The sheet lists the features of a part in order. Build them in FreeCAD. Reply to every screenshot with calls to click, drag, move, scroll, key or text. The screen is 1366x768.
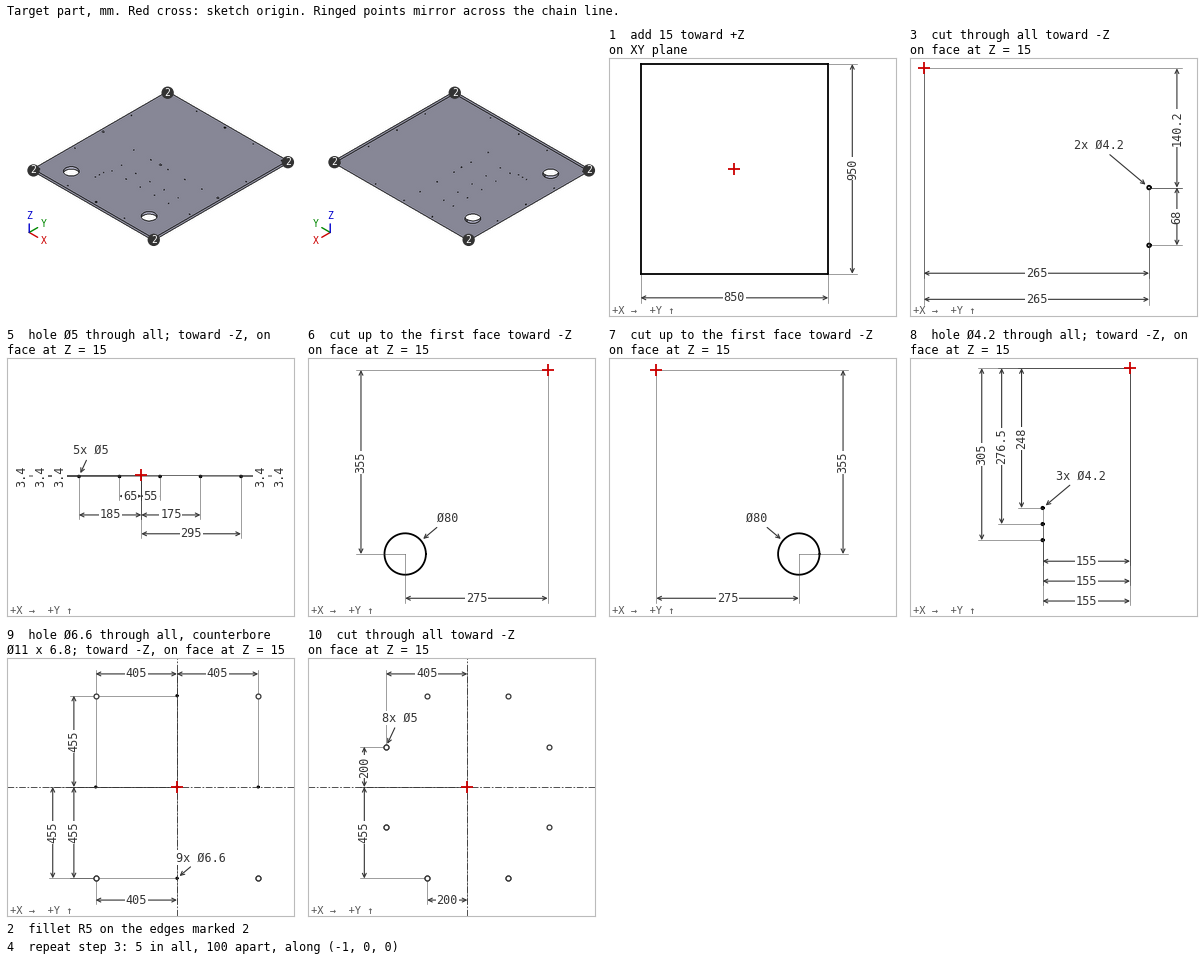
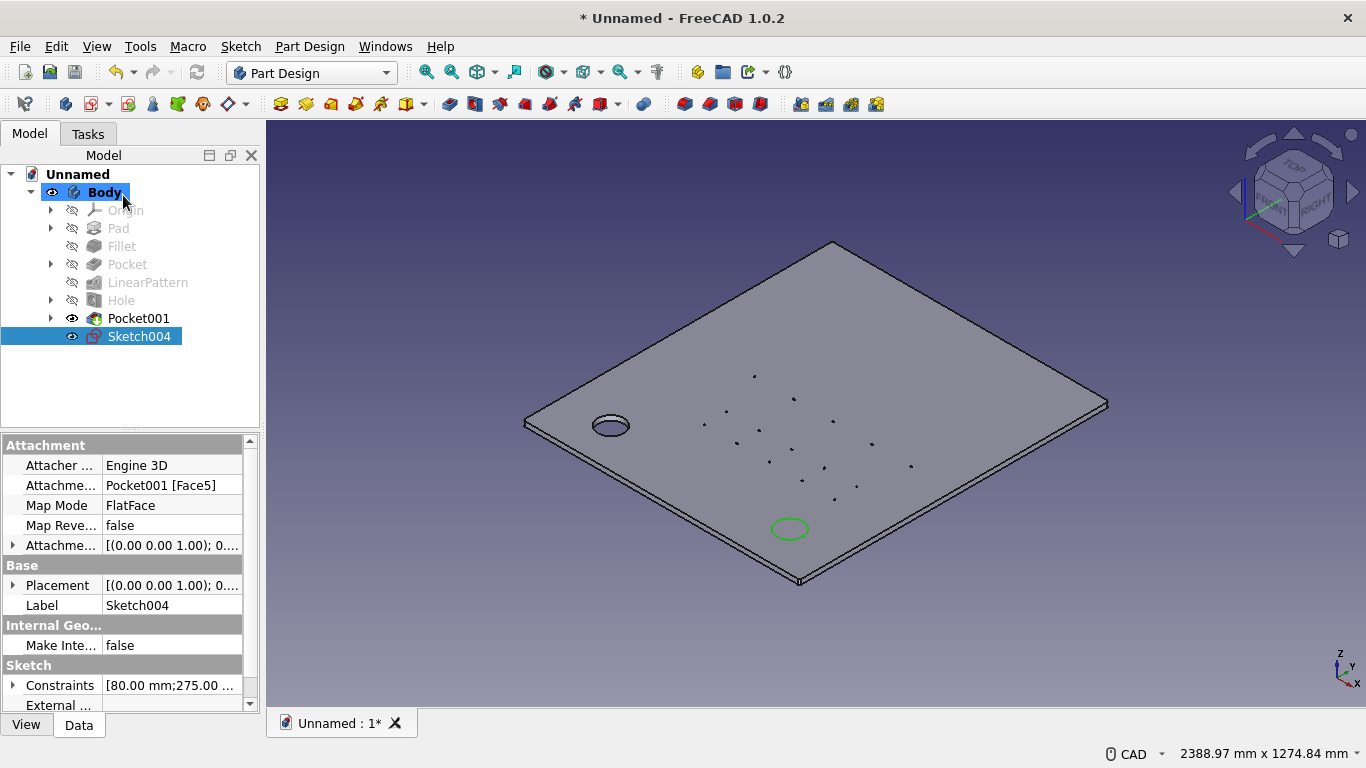
click(450, 104)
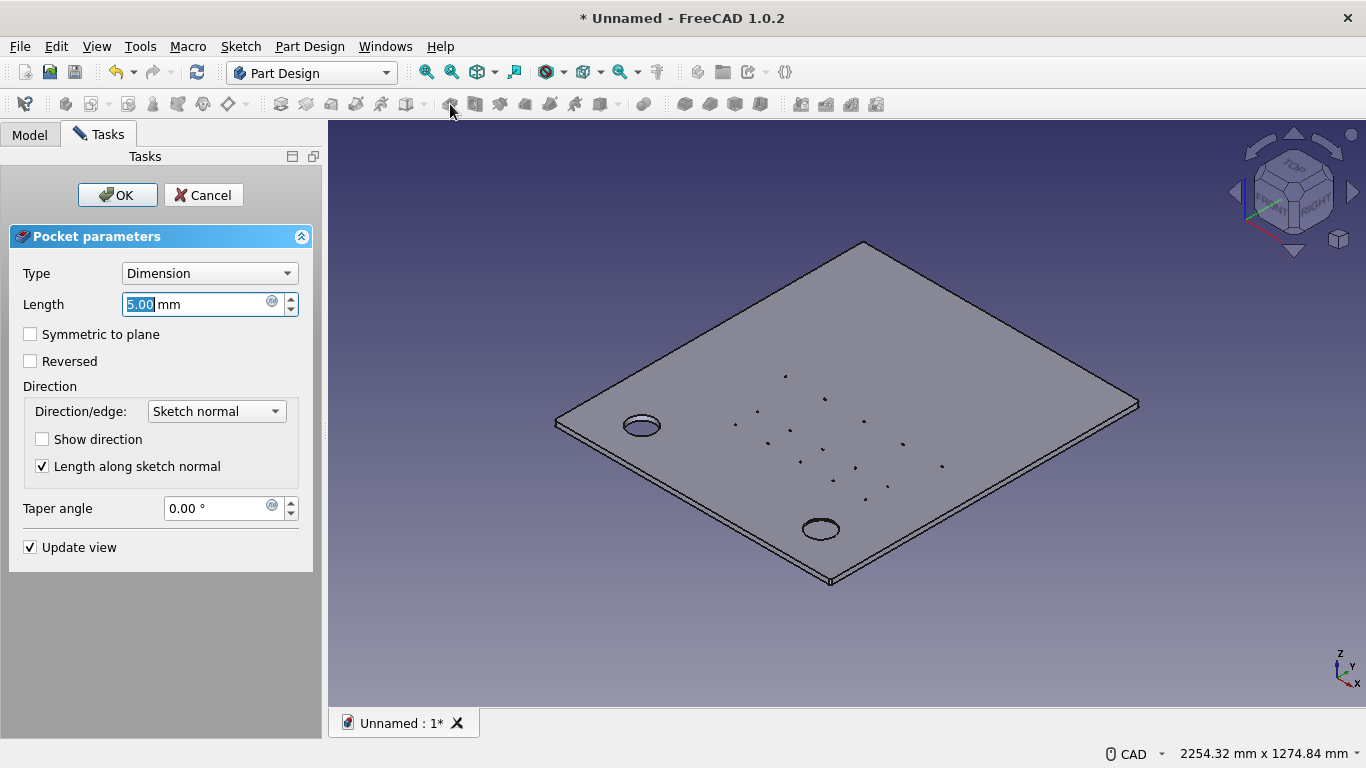
click(210, 274)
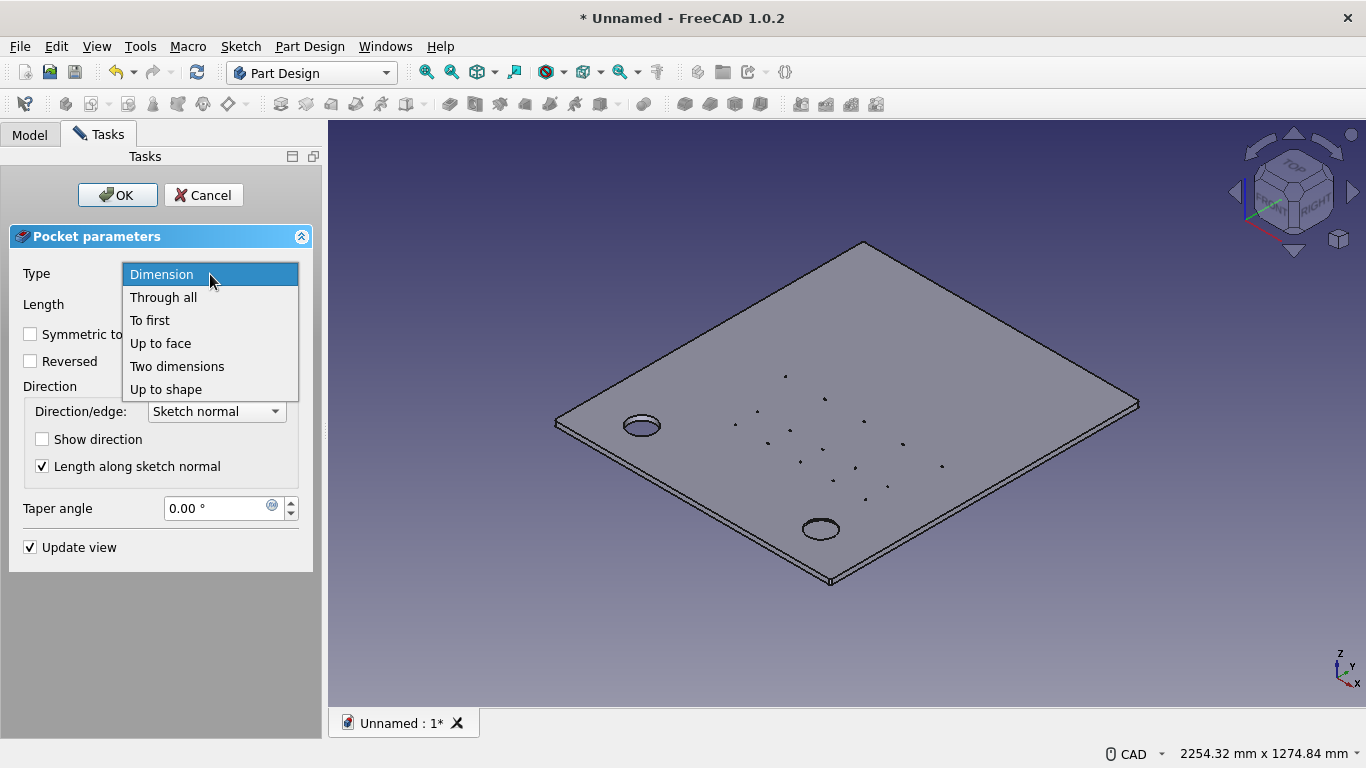
click(208, 320)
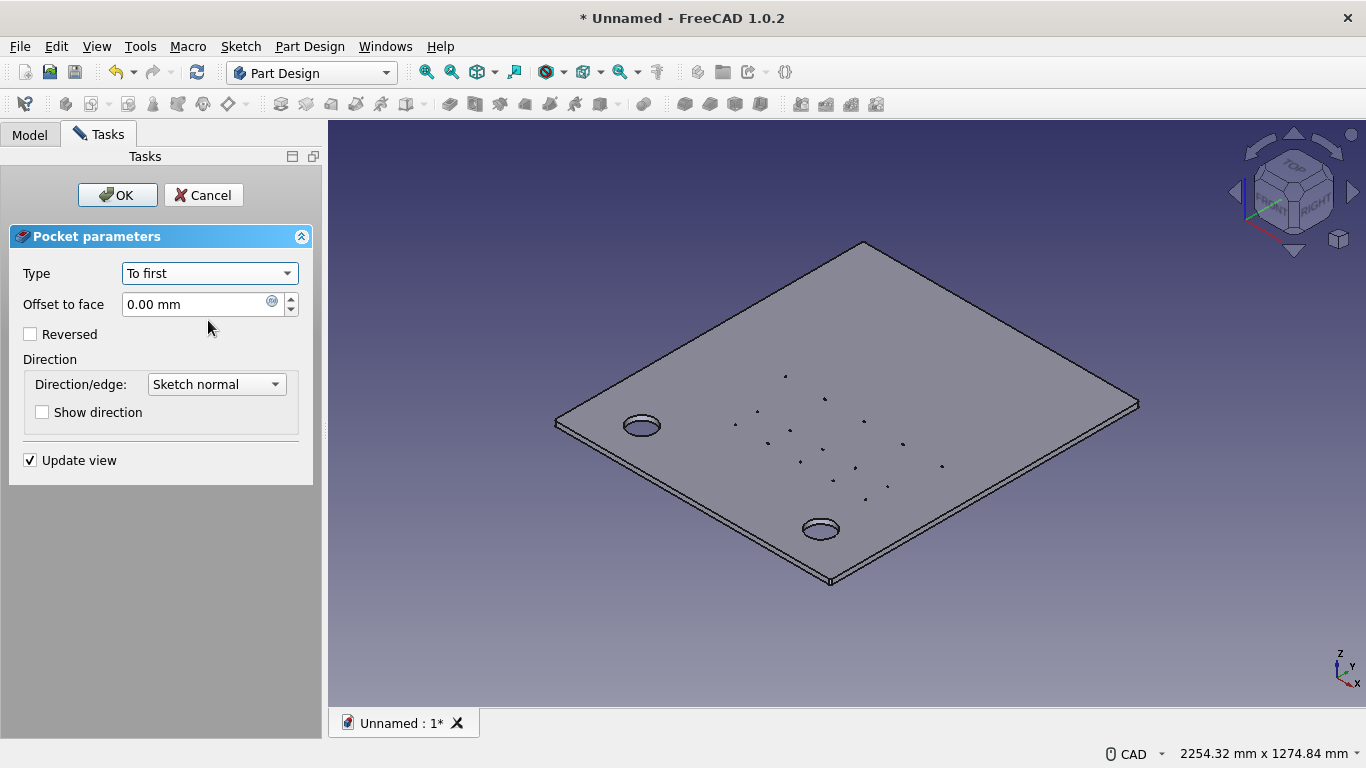
click(118, 195)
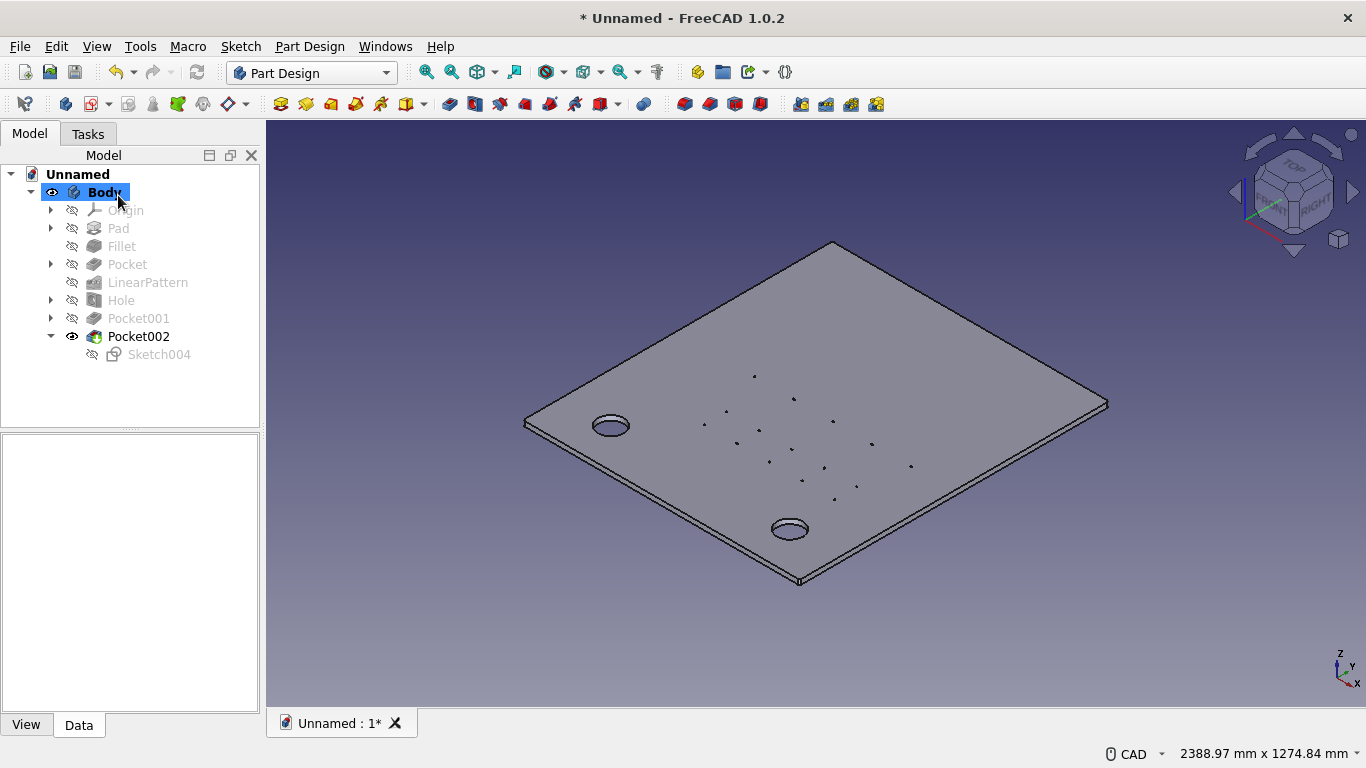
click(944, 381)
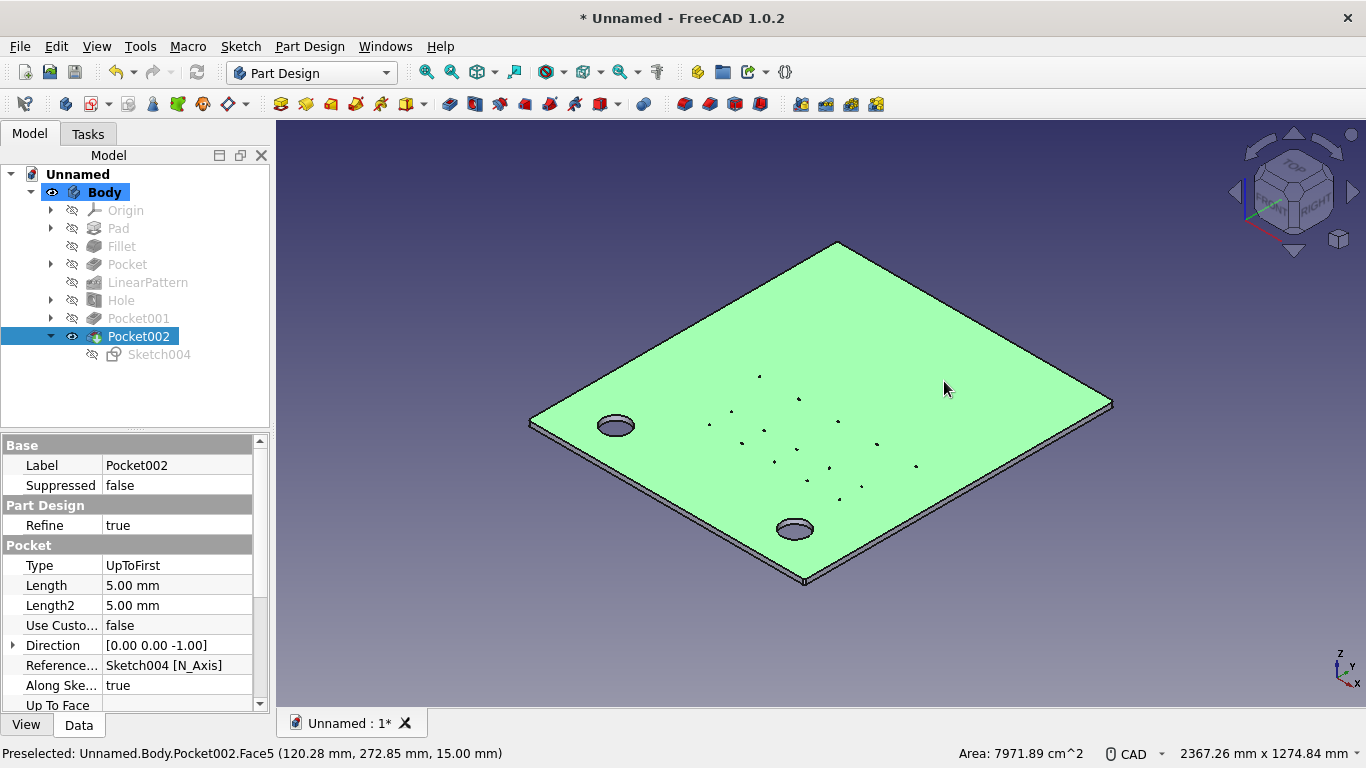
click(90, 104)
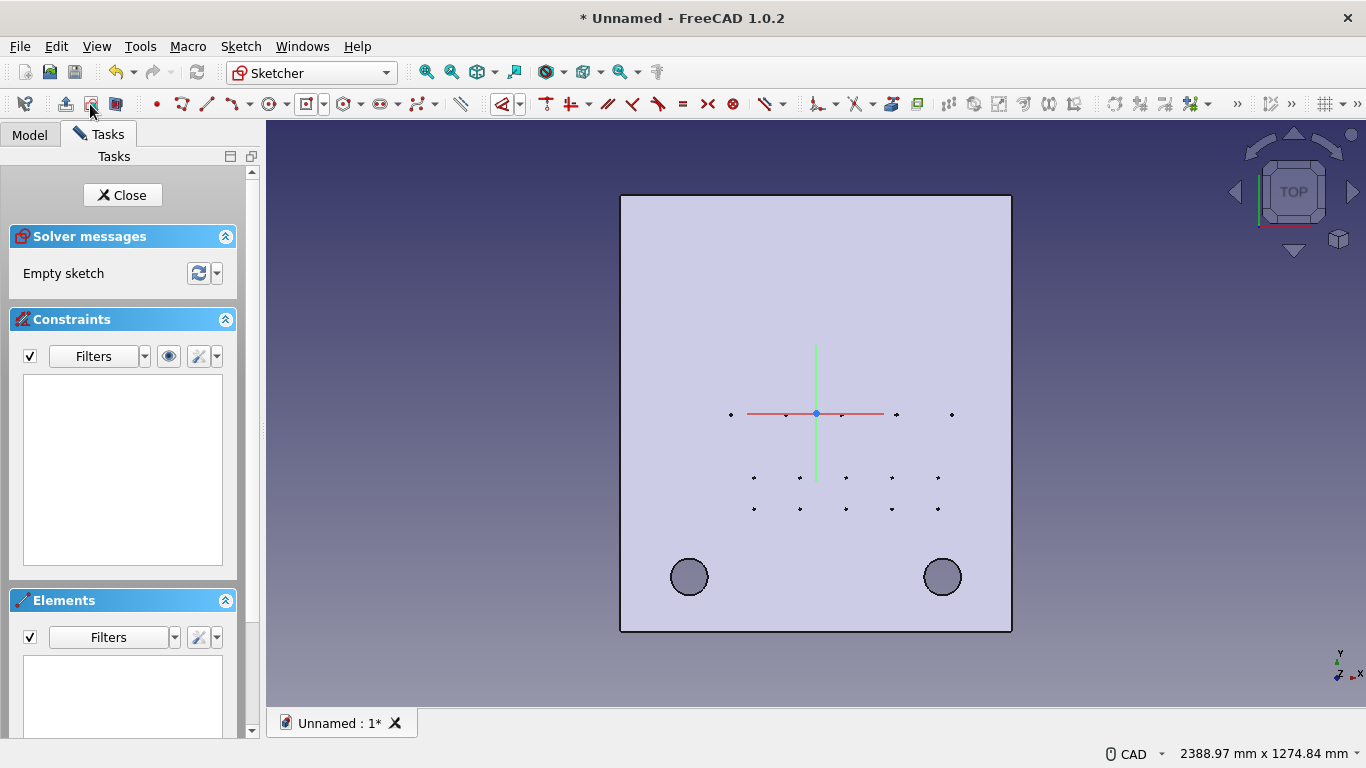
scroll(744, 551, up, 13)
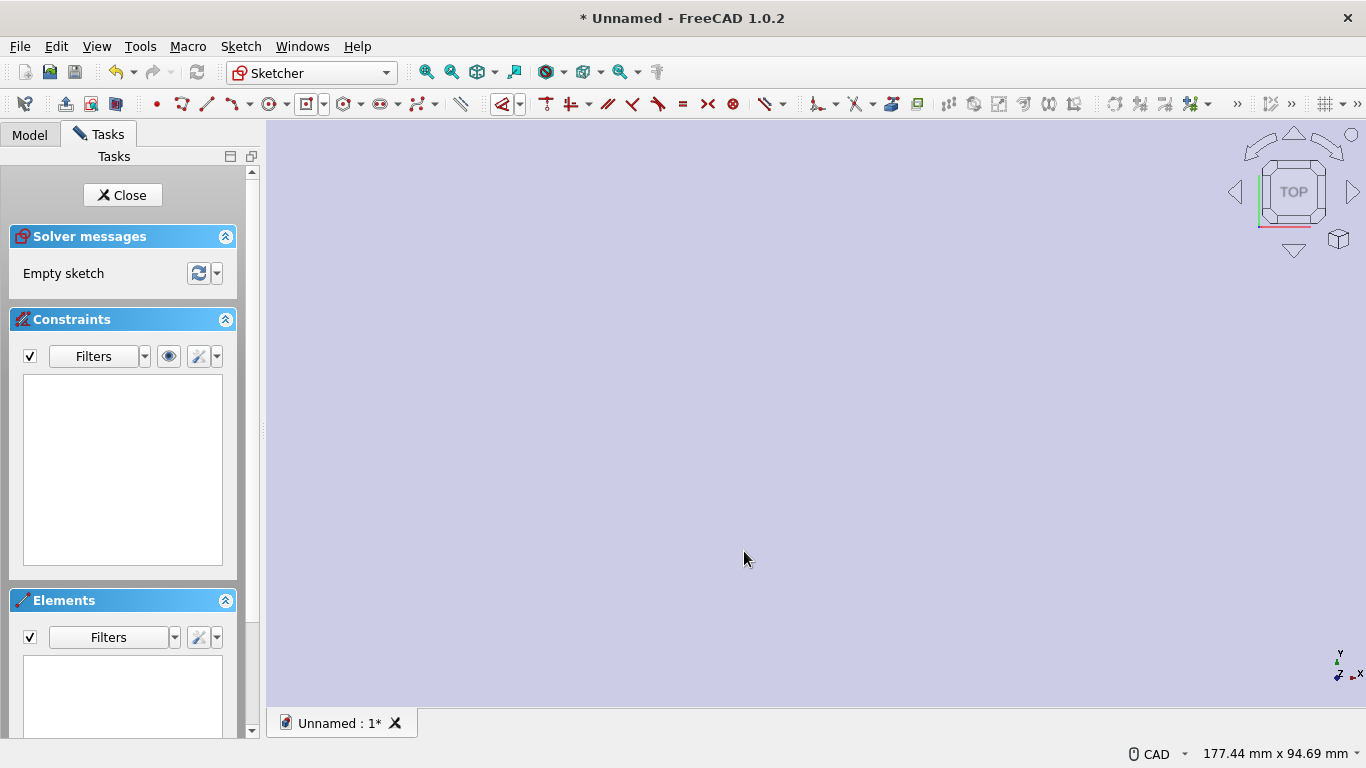
click(268, 104)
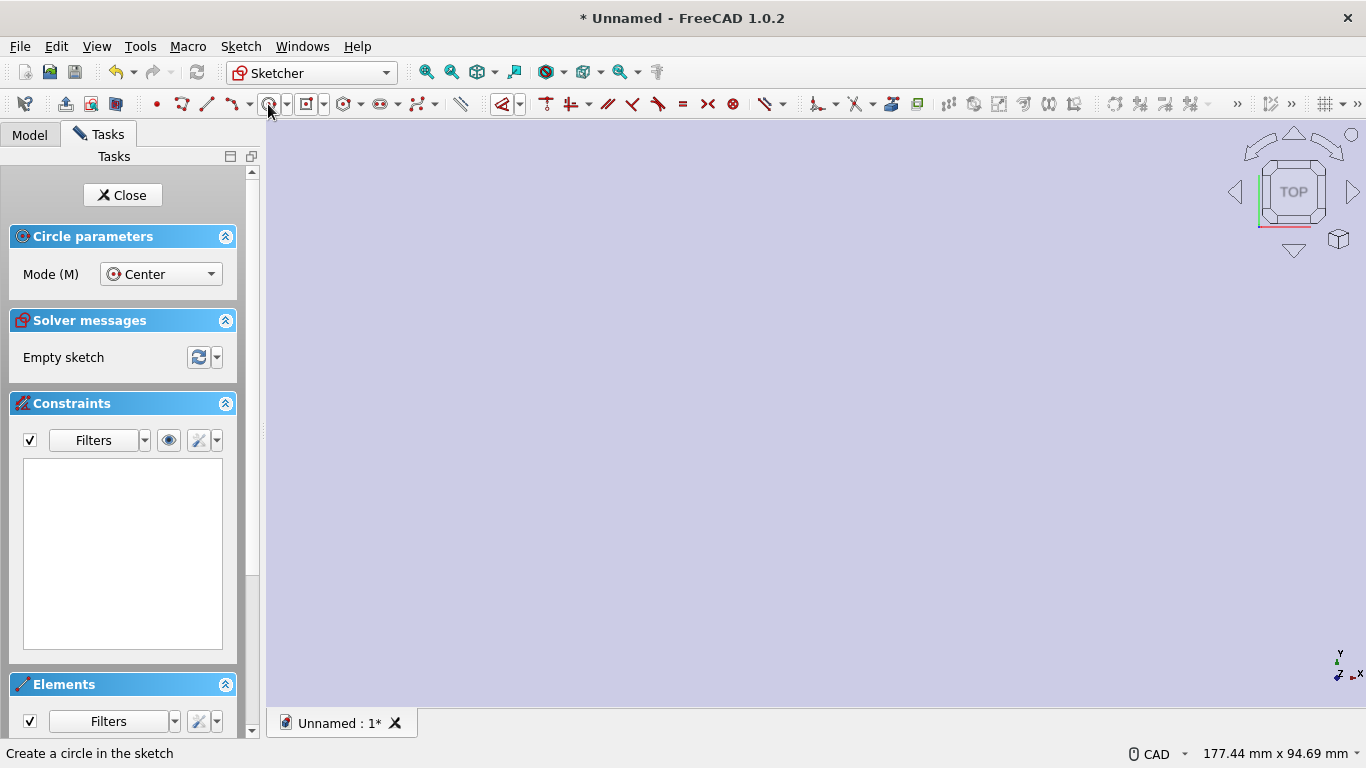
scroll(747, 228, up, 3)